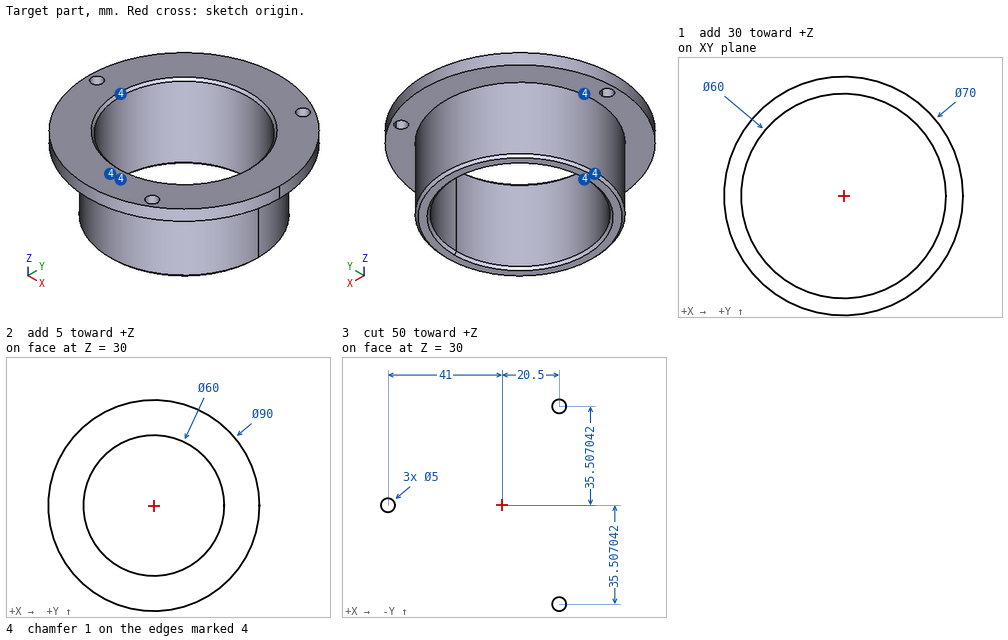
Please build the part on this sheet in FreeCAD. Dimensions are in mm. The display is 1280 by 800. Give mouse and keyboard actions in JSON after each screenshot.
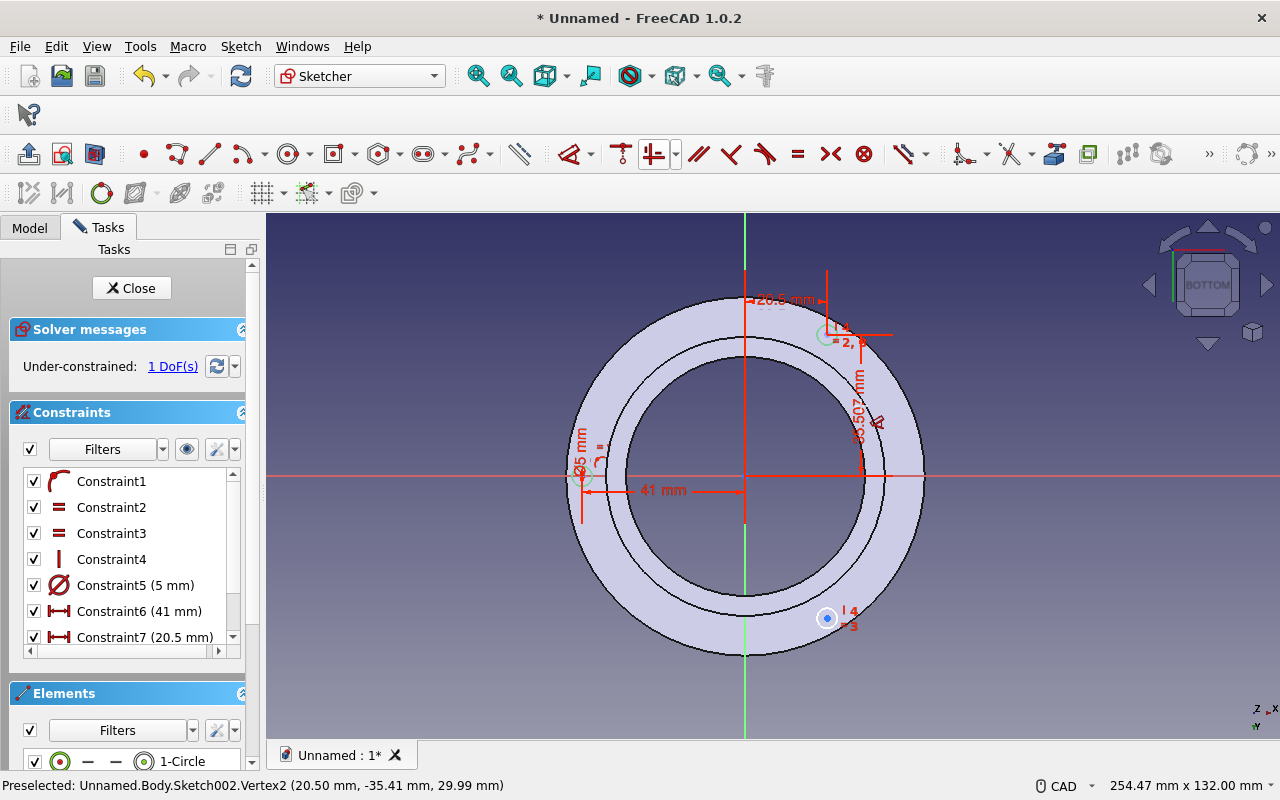
{"action": "left_click", "coordinate": [827, 618]}
{"action": "left_click", "coordinate": [861, 547]}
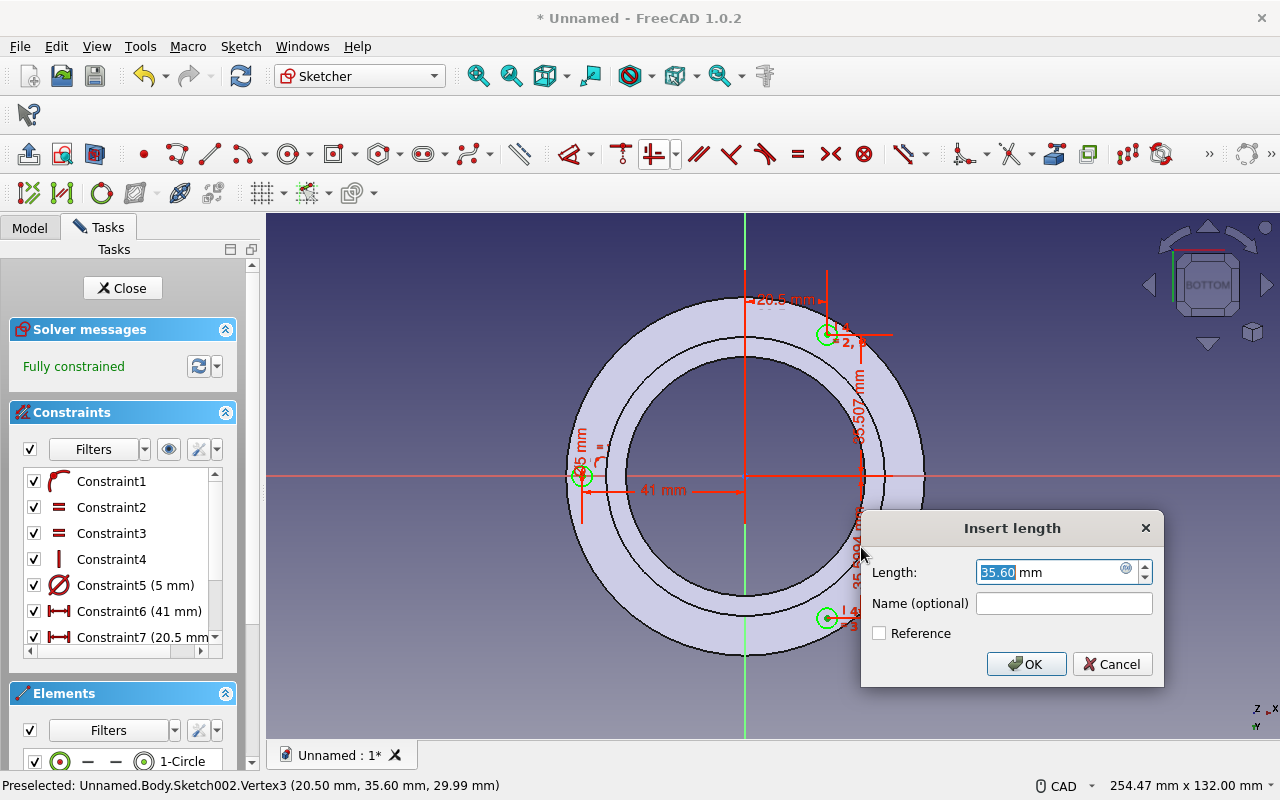
{"action": "type", "text": "35.507042"}
{"action": "key", "text": "Return"}
{"action": "key", "text": "Escape"}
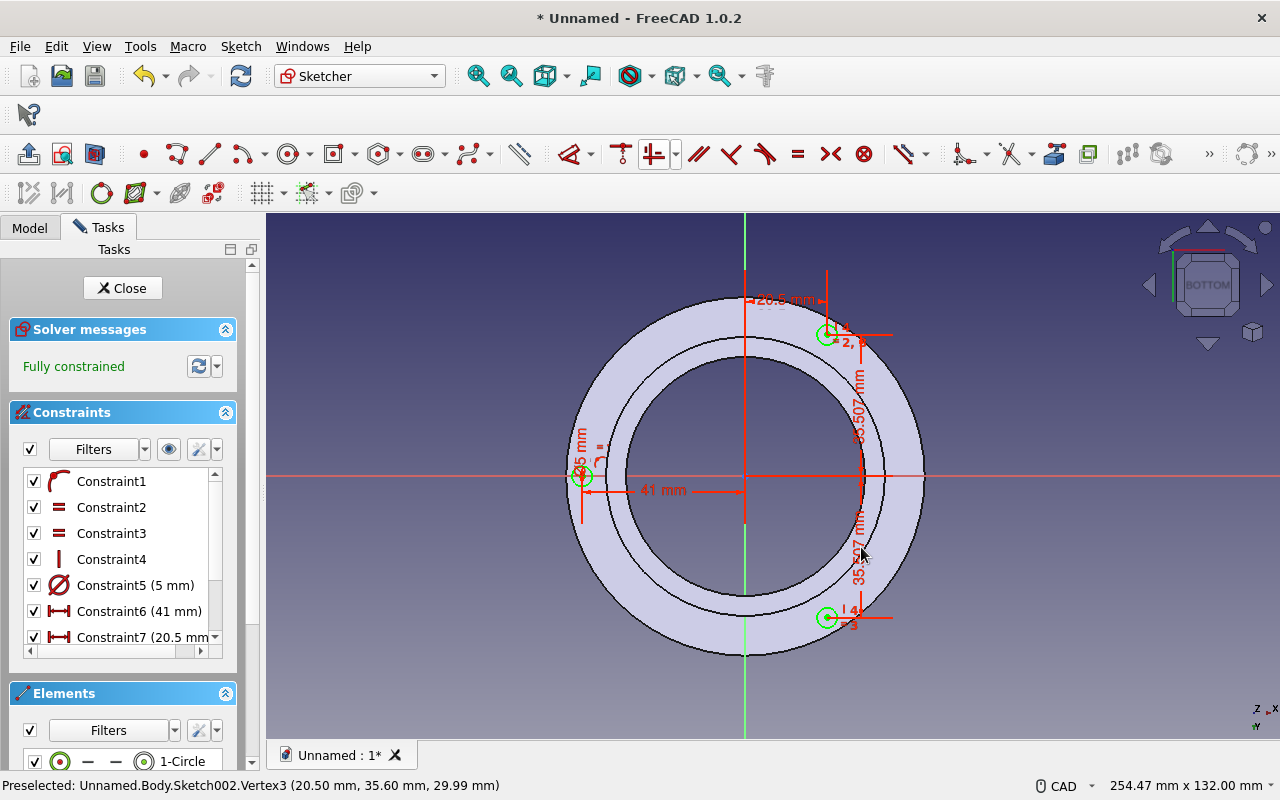
{"action": "left_click", "coordinate": [123, 288]}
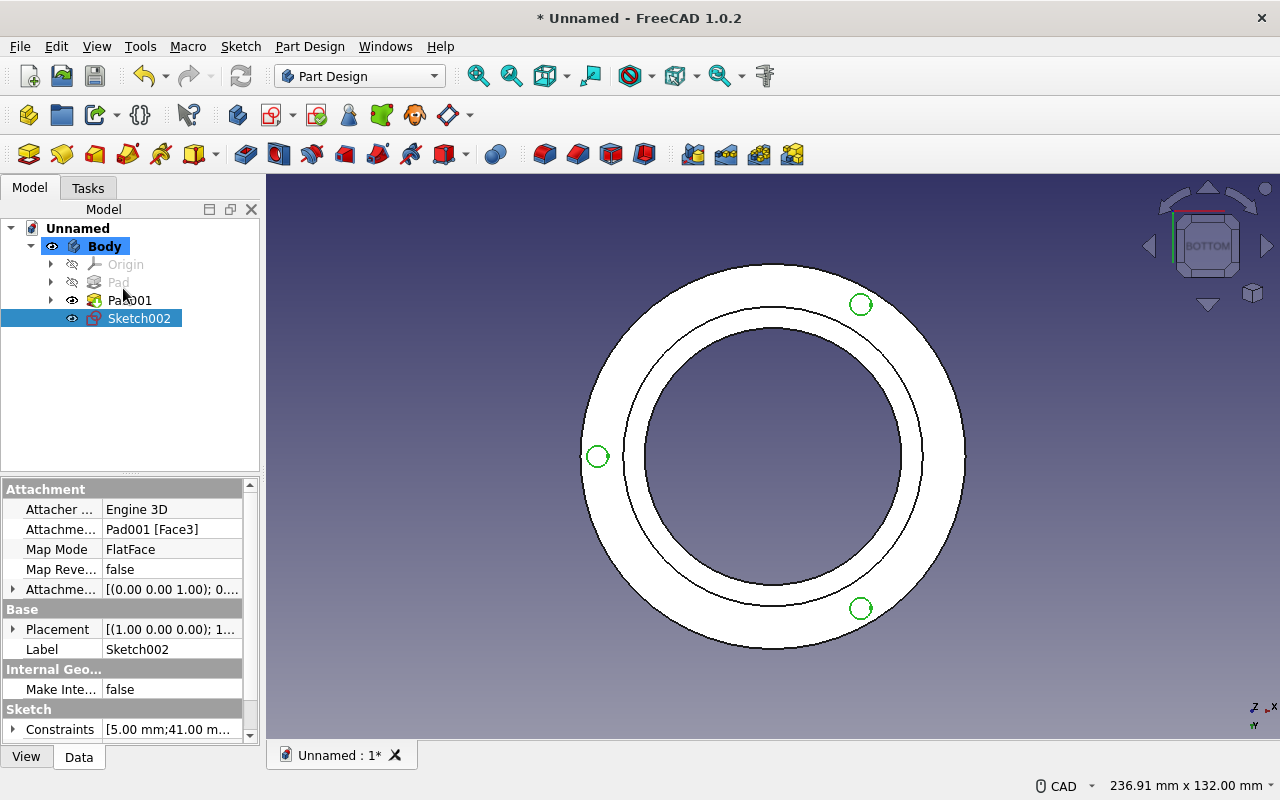
{"action": "left_click", "coordinate": [246, 154]}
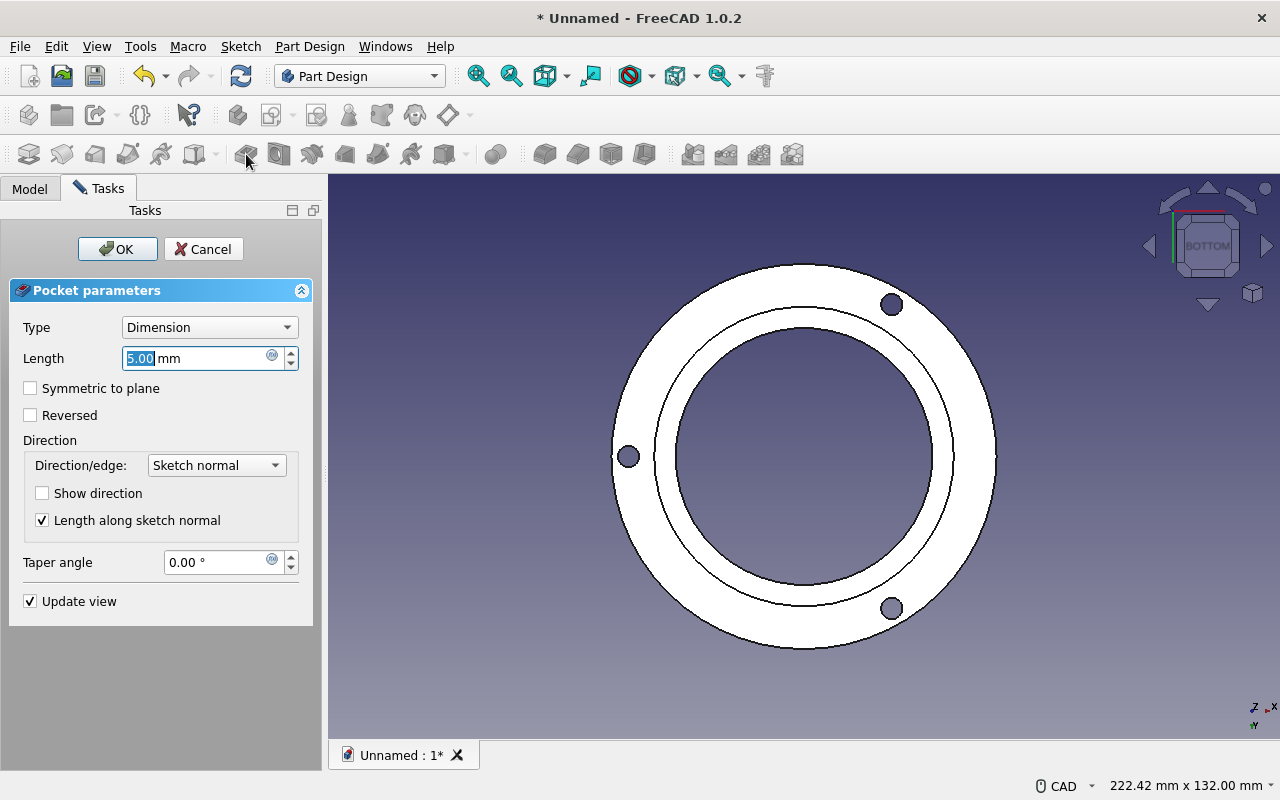
{"action": "type", "text": "50"}
{"action": "key", "text": "Tab"}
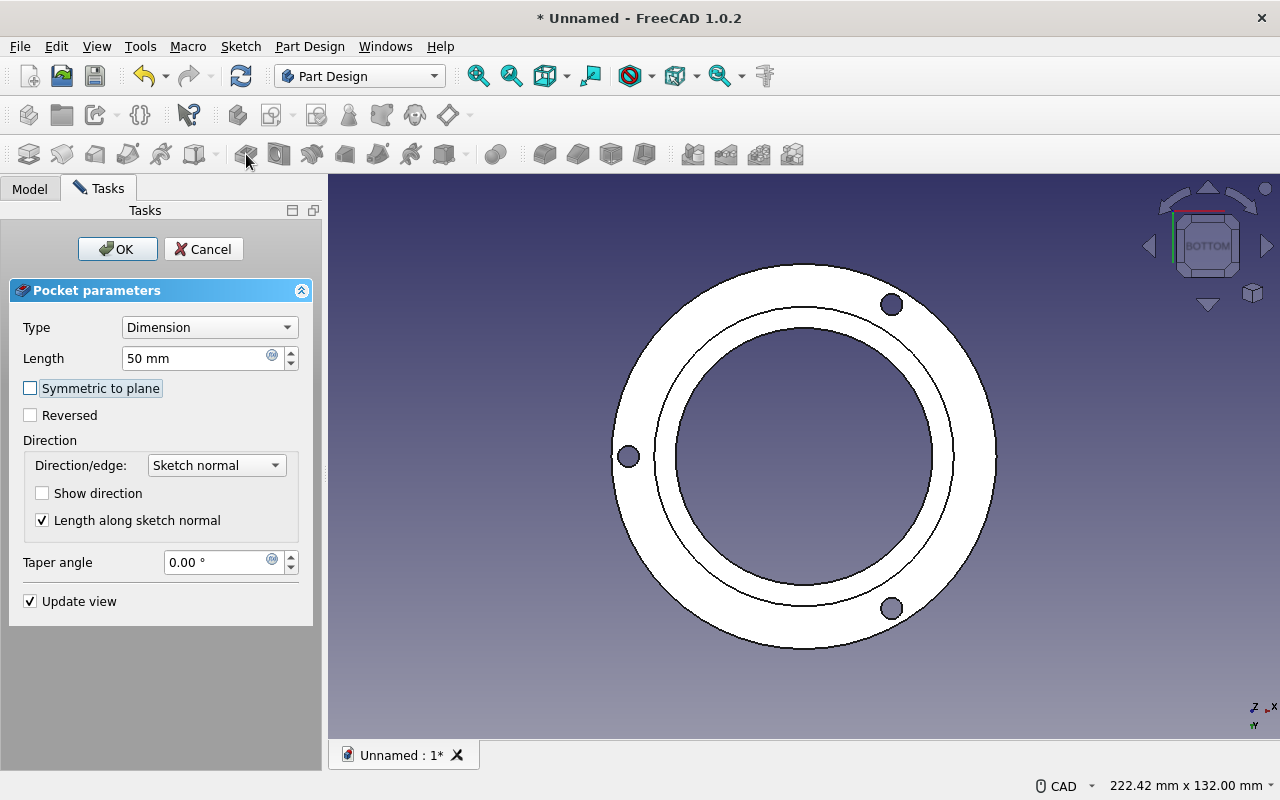
{"action": "left_click", "coordinate": [118, 249]}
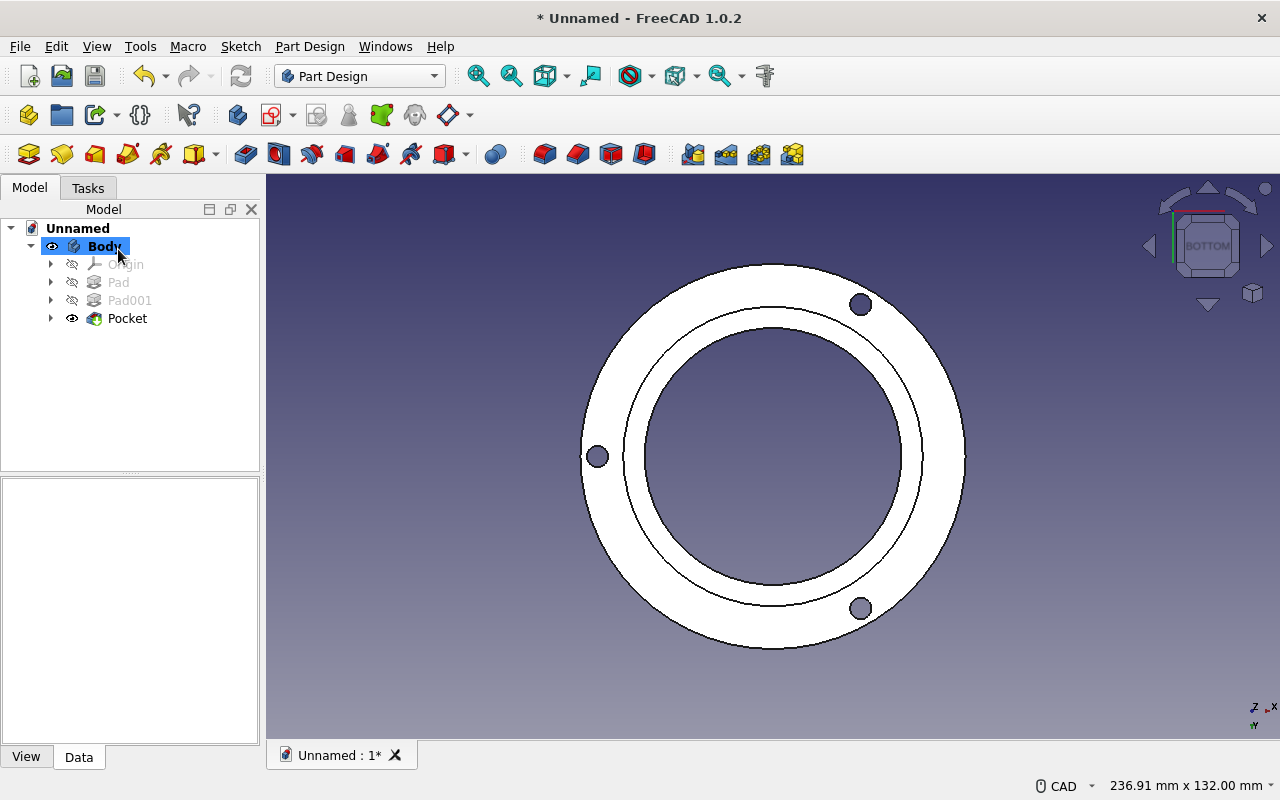
{"action": "left_click", "coordinate": [623, 456]}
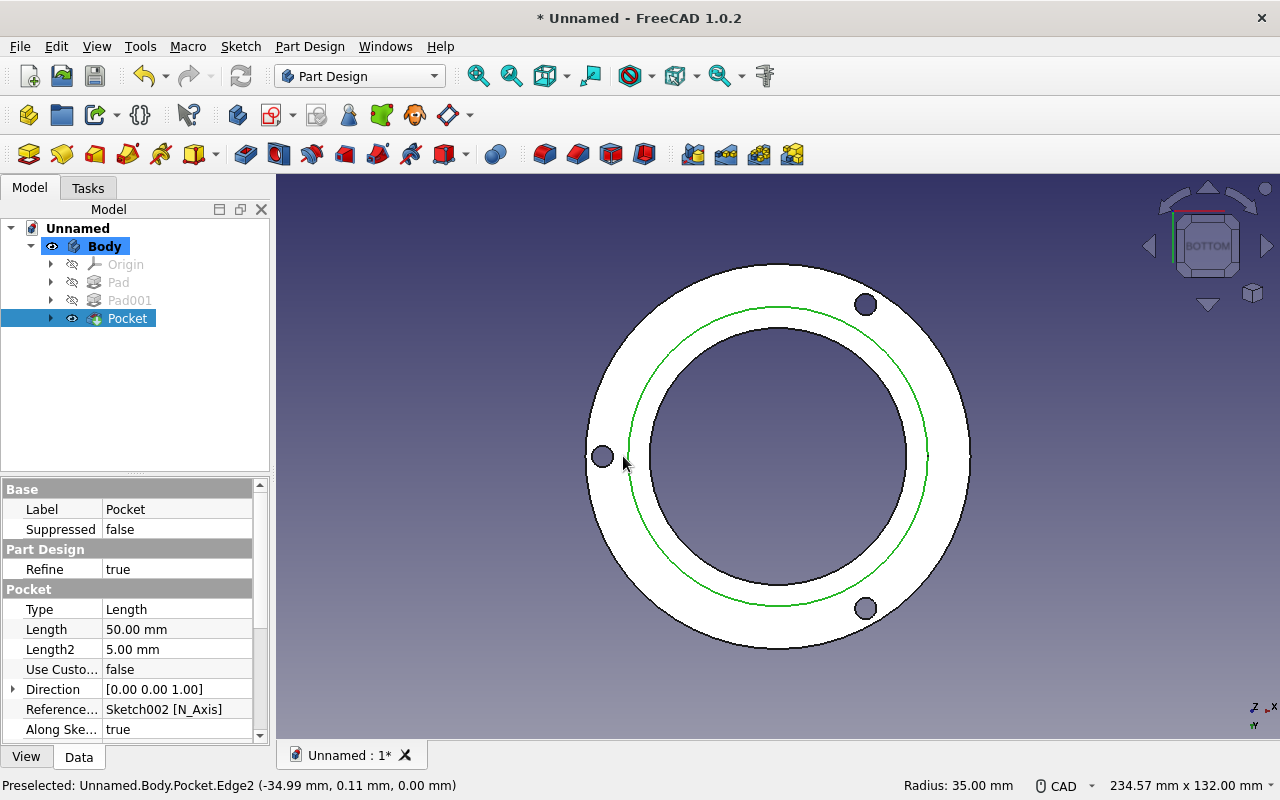
{"action": "left_click", "coordinate": [674, 380], "text": "ctrl"}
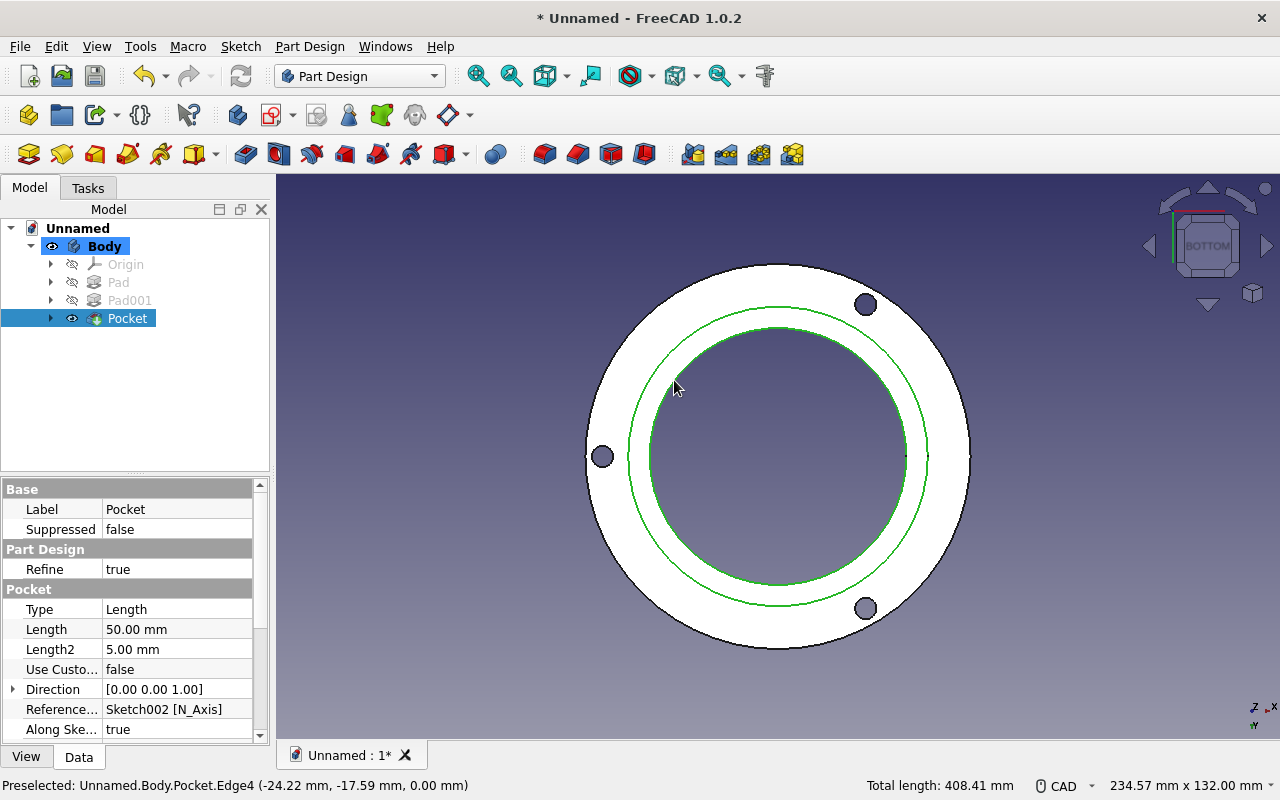
{"action": "key", "text": "0"}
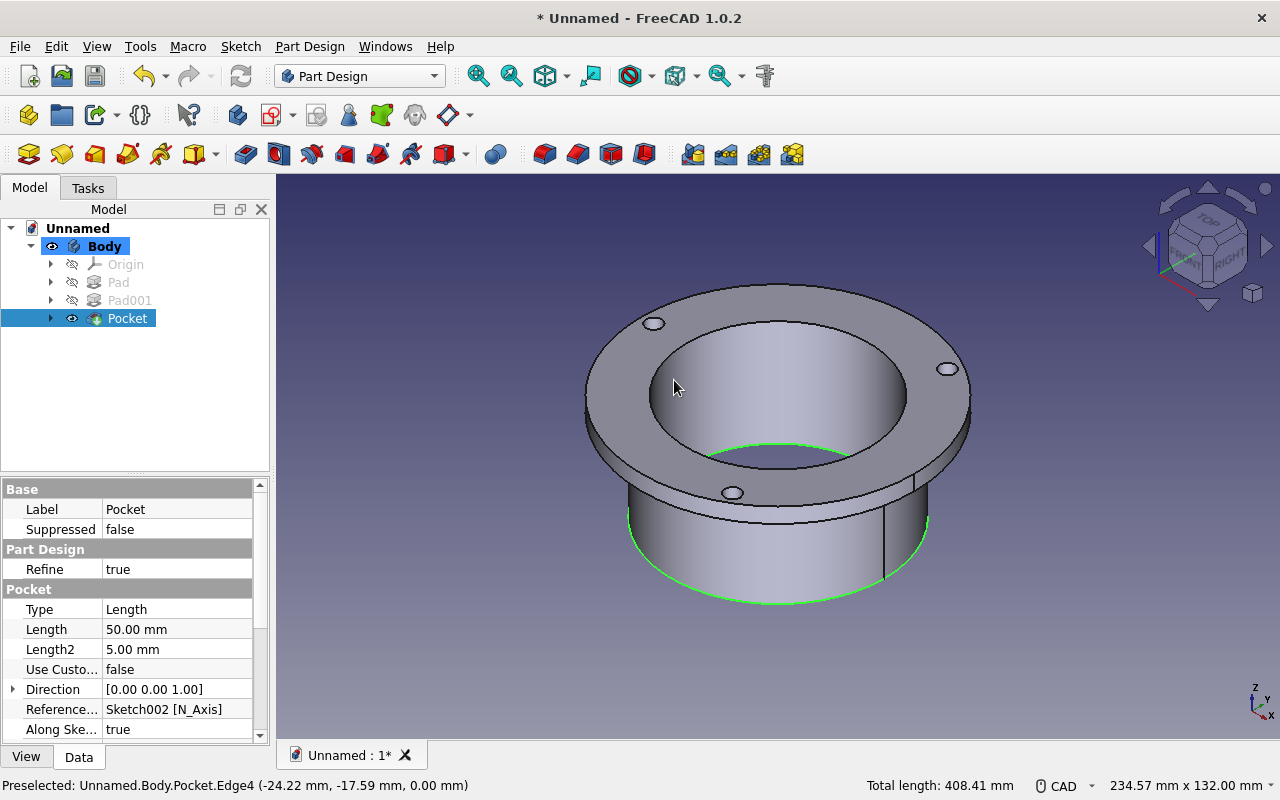
{"action": "left_click", "coordinate": [687, 342], "text": "ctrl"}